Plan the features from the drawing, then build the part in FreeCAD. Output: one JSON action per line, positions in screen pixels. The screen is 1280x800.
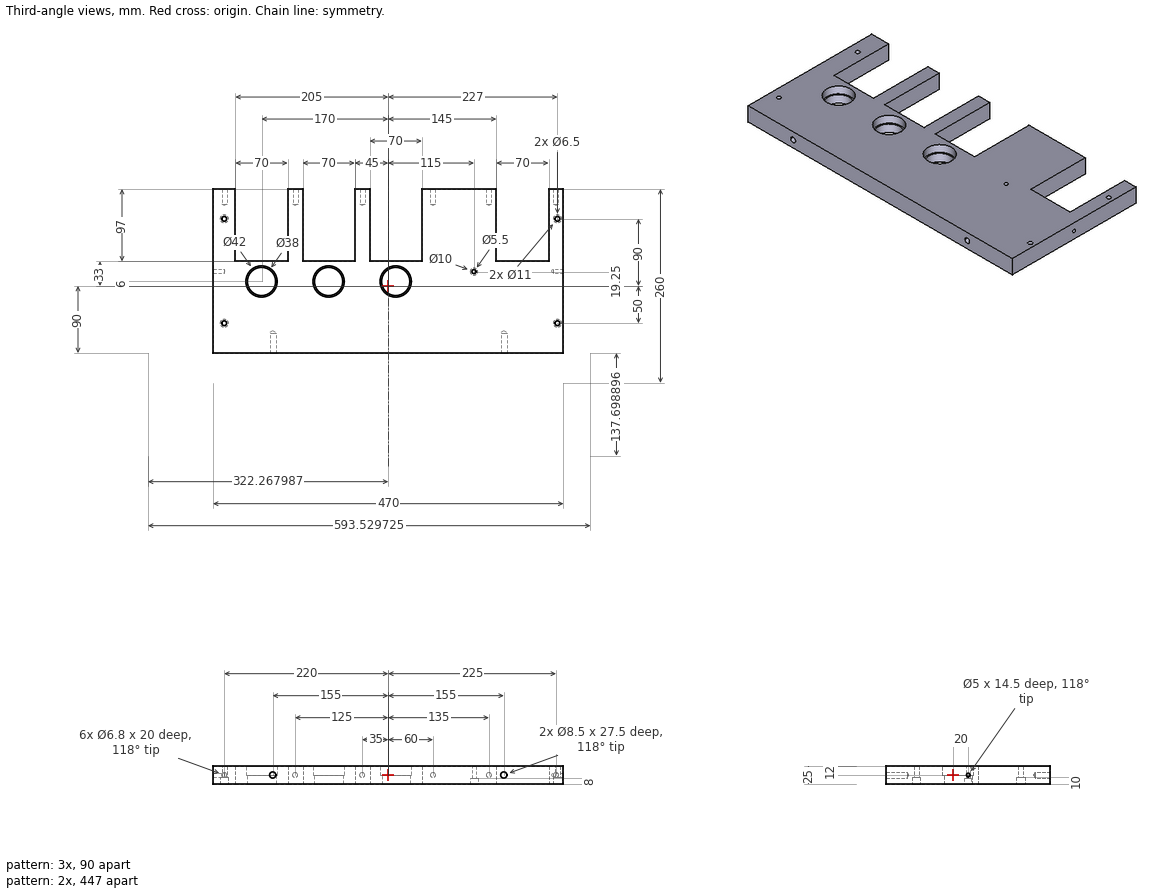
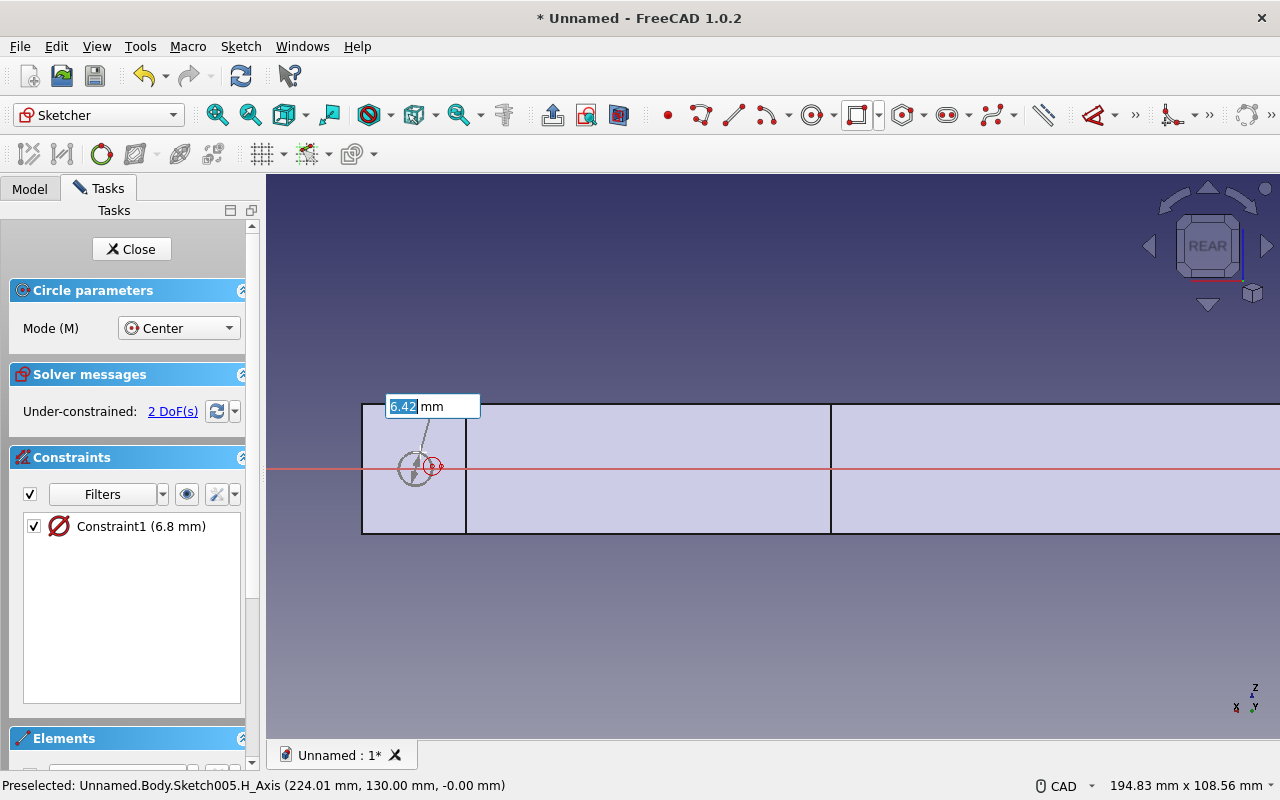
{"action": "type", "text": "6.8"}
{"action": "key", "text": "Return"}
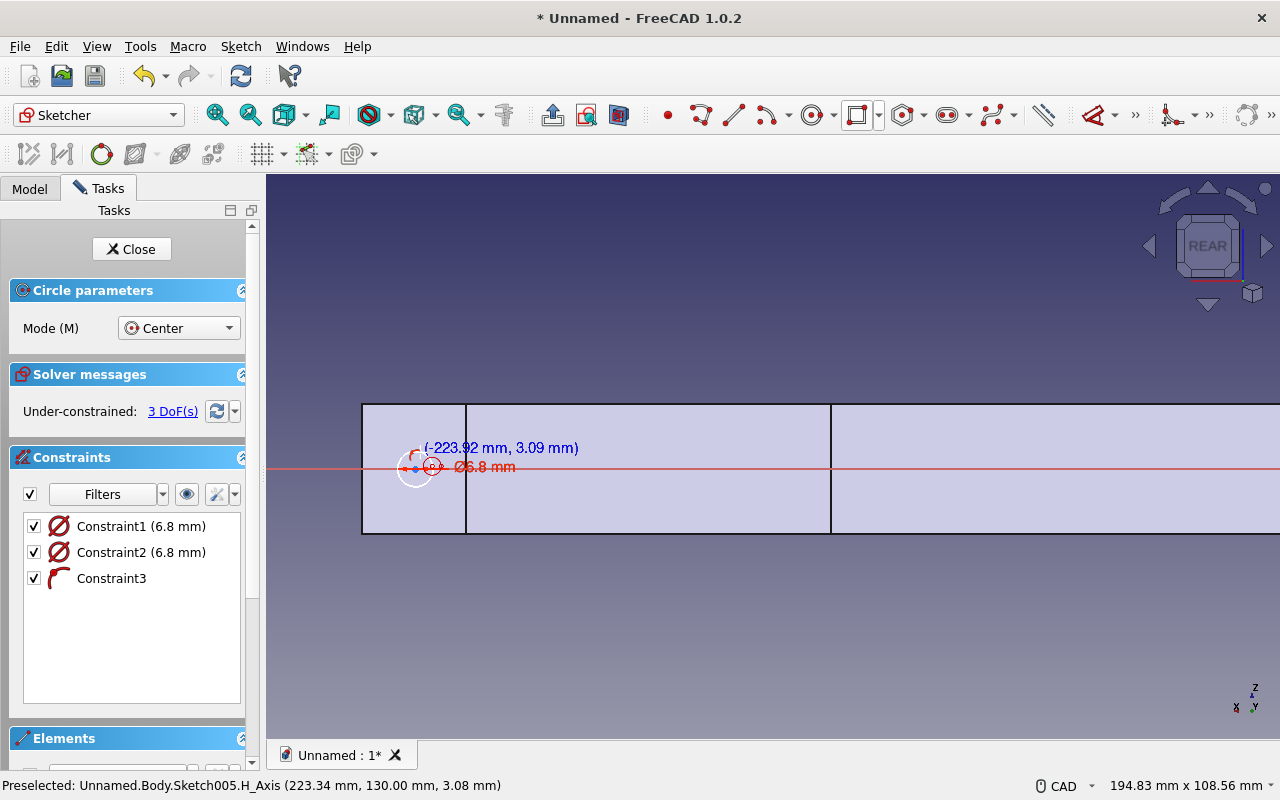
{"action": "scroll", "coordinate": [883, 469], "scroll_direction": "up", "scroll_amount": 2}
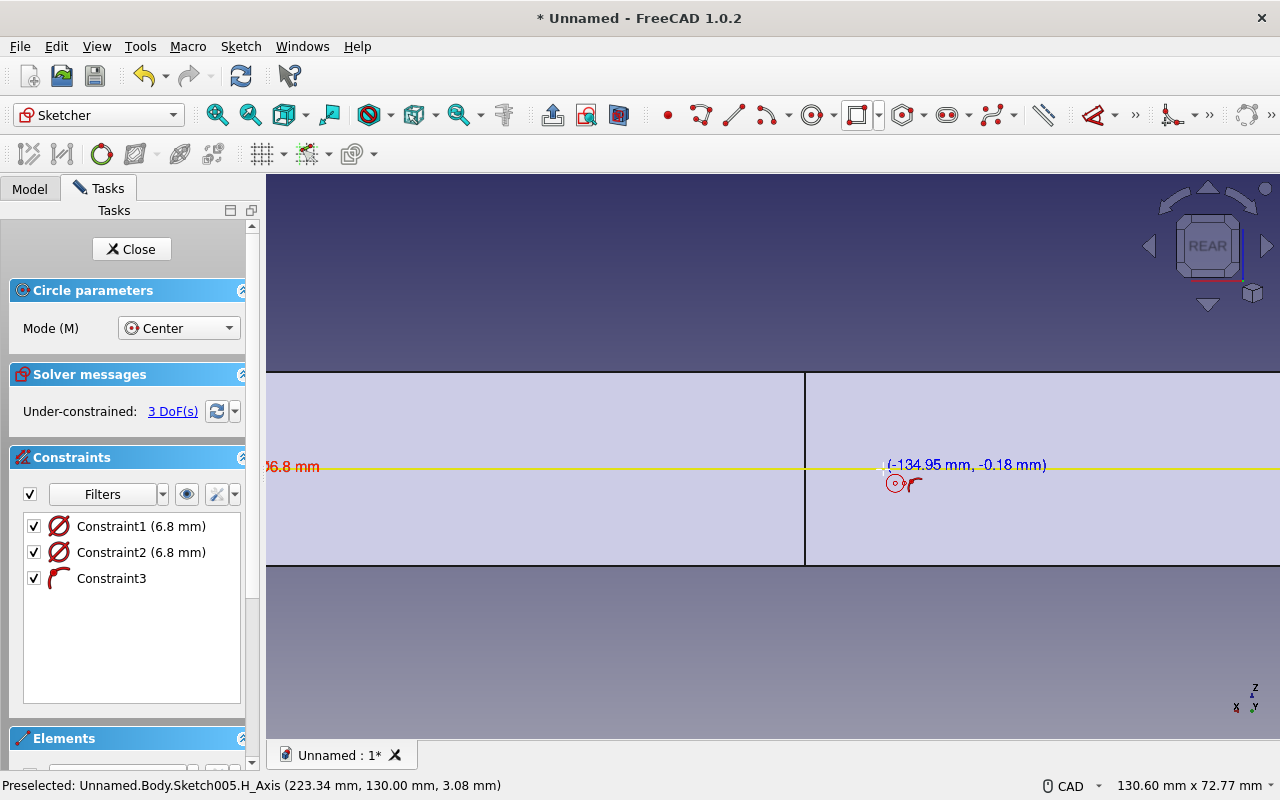
{"action": "scroll", "coordinate": [466, 454], "scroll_direction": "down", "scroll_amount": 9}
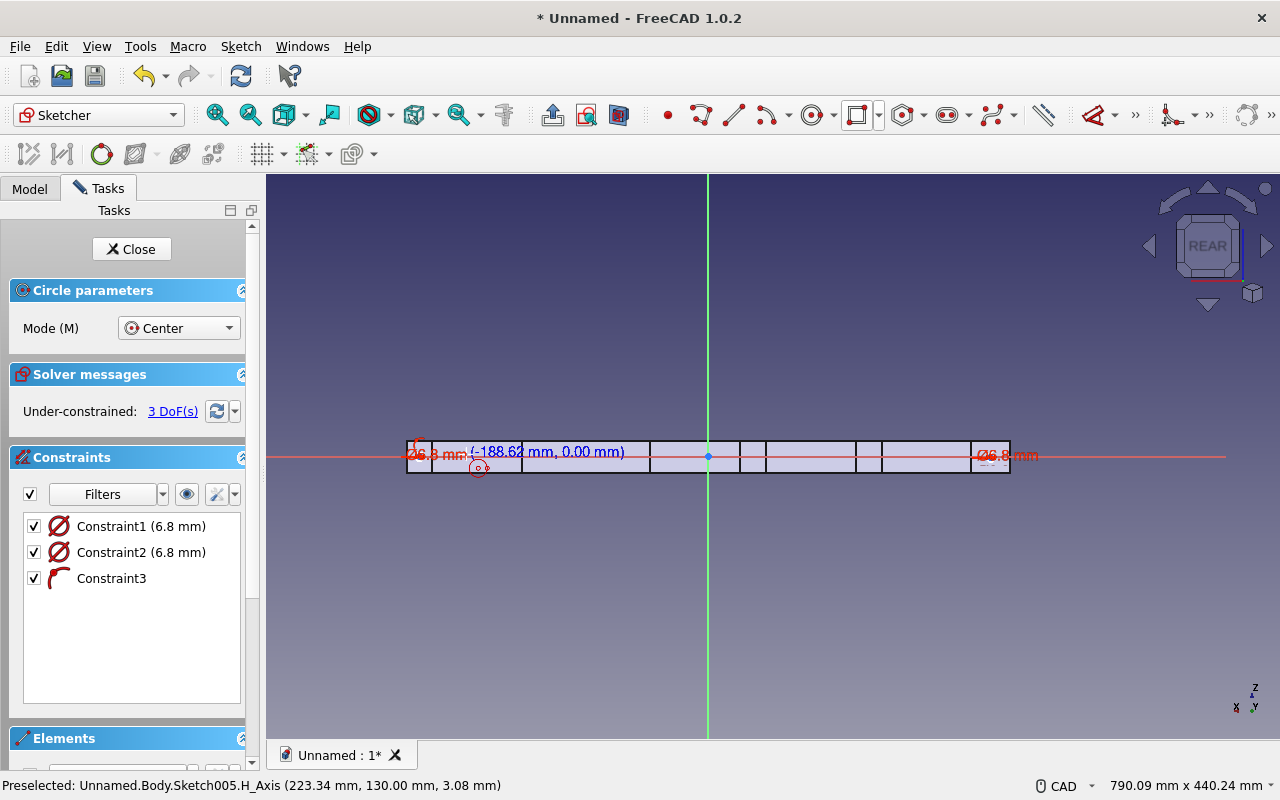
{"action": "left_click", "coordinate": [535, 457]}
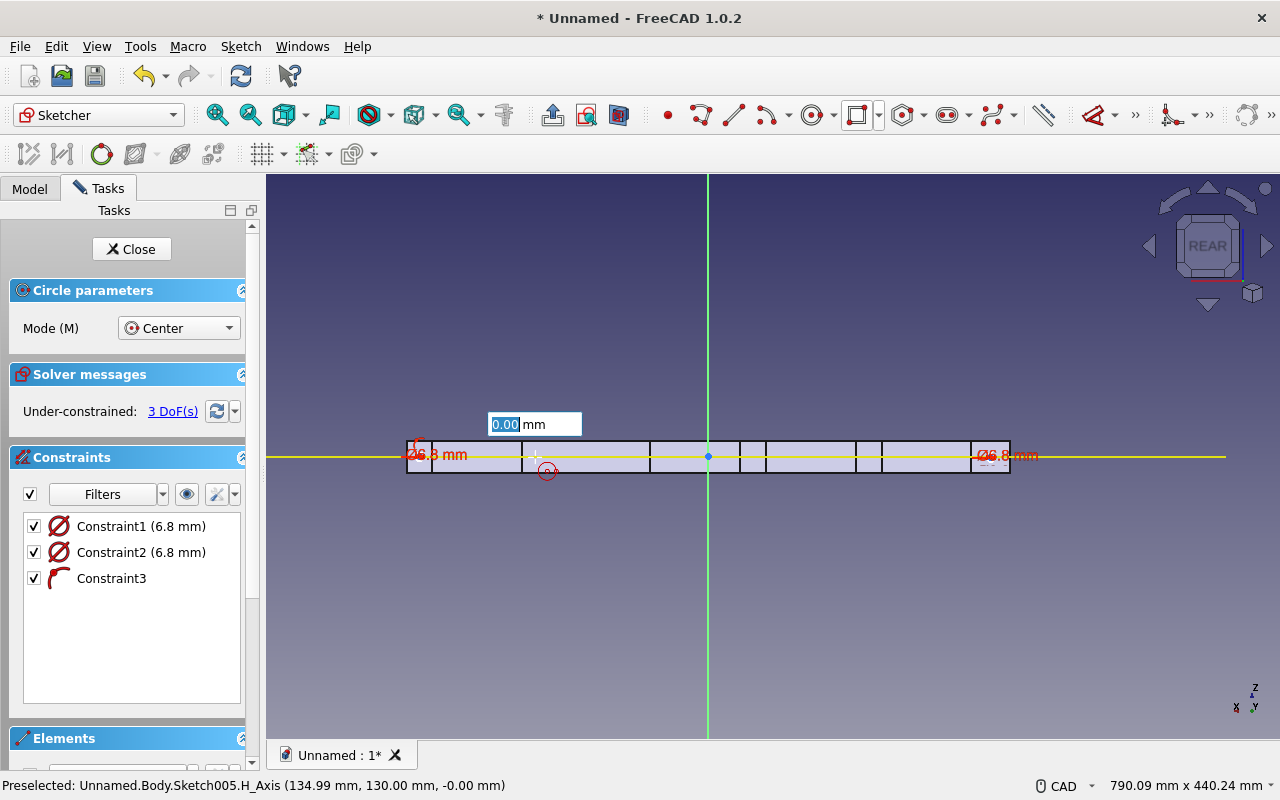
{"action": "scroll", "coordinate": [533, 461], "scroll_direction": "up", "scroll_amount": 7}
{"action": "mouse_move", "coordinate": [534, 459]}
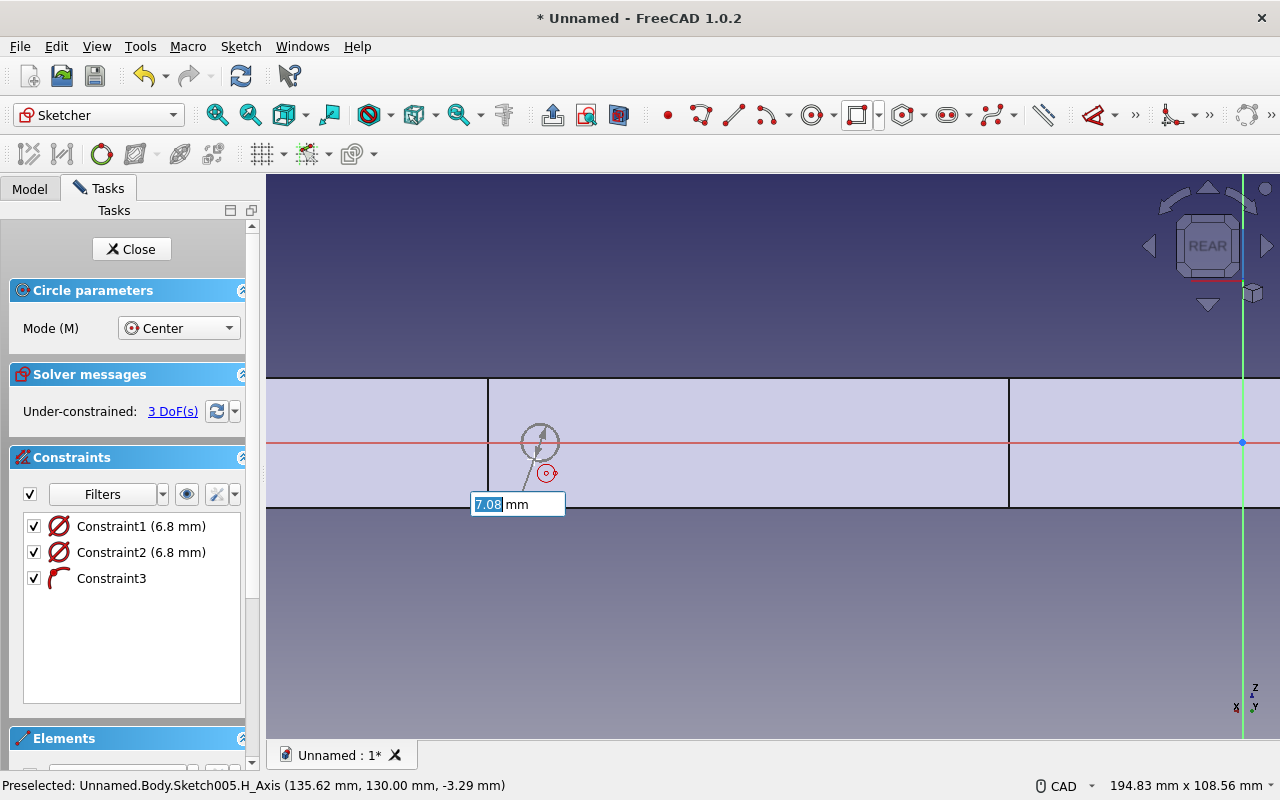
{"action": "type", "text": "6.8"}
{"action": "key", "text": "Return"}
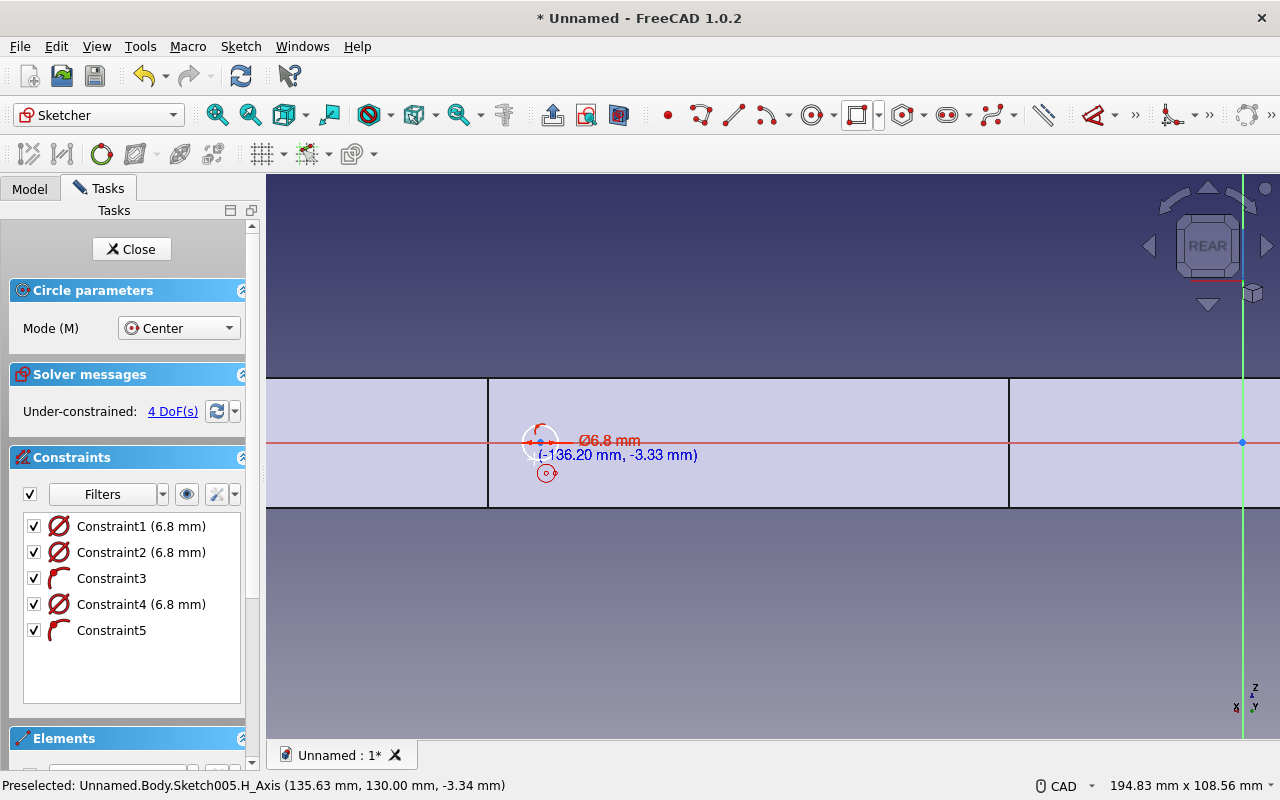
{"action": "scroll", "coordinate": [533, 461], "scroll_direction": "down", "scroll_amount": 7}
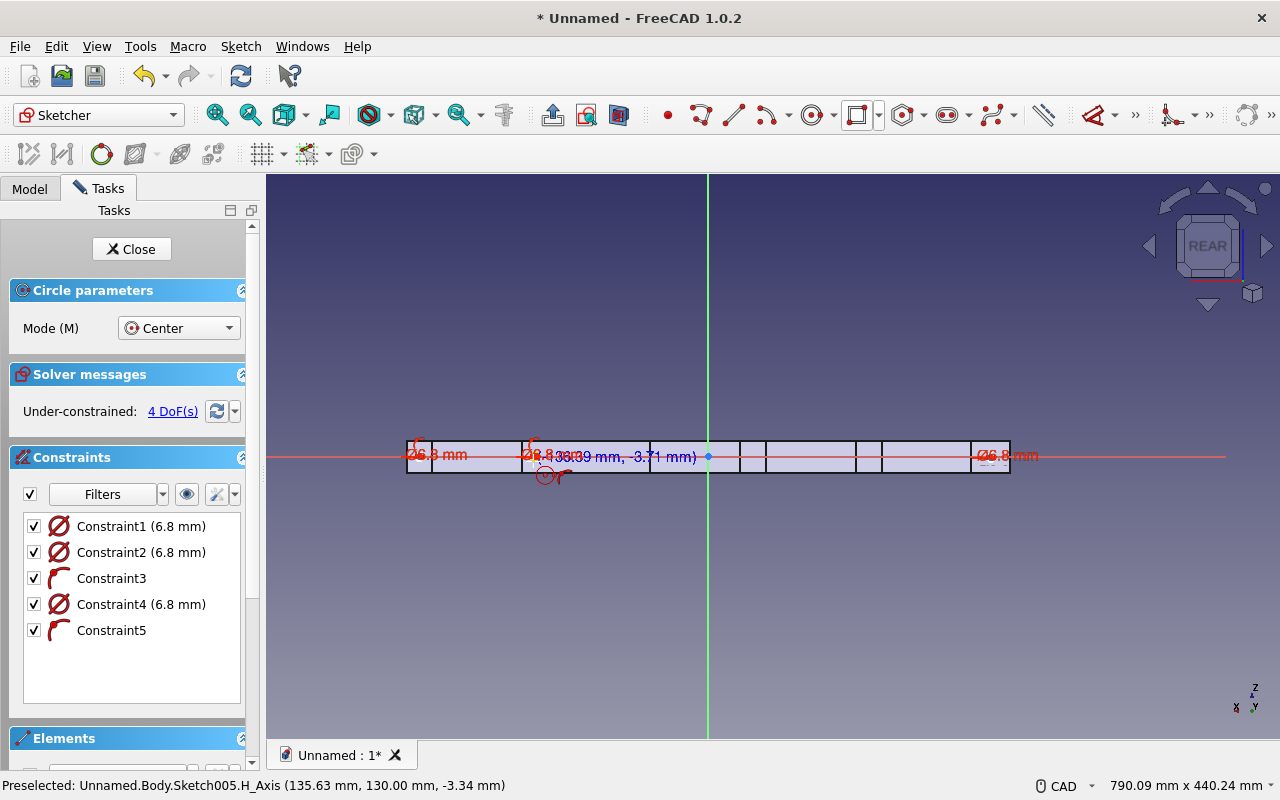
{"action": "scroll", "coordinate": [753, 457], "scroll_direction": "up", "scroll_amount": 9}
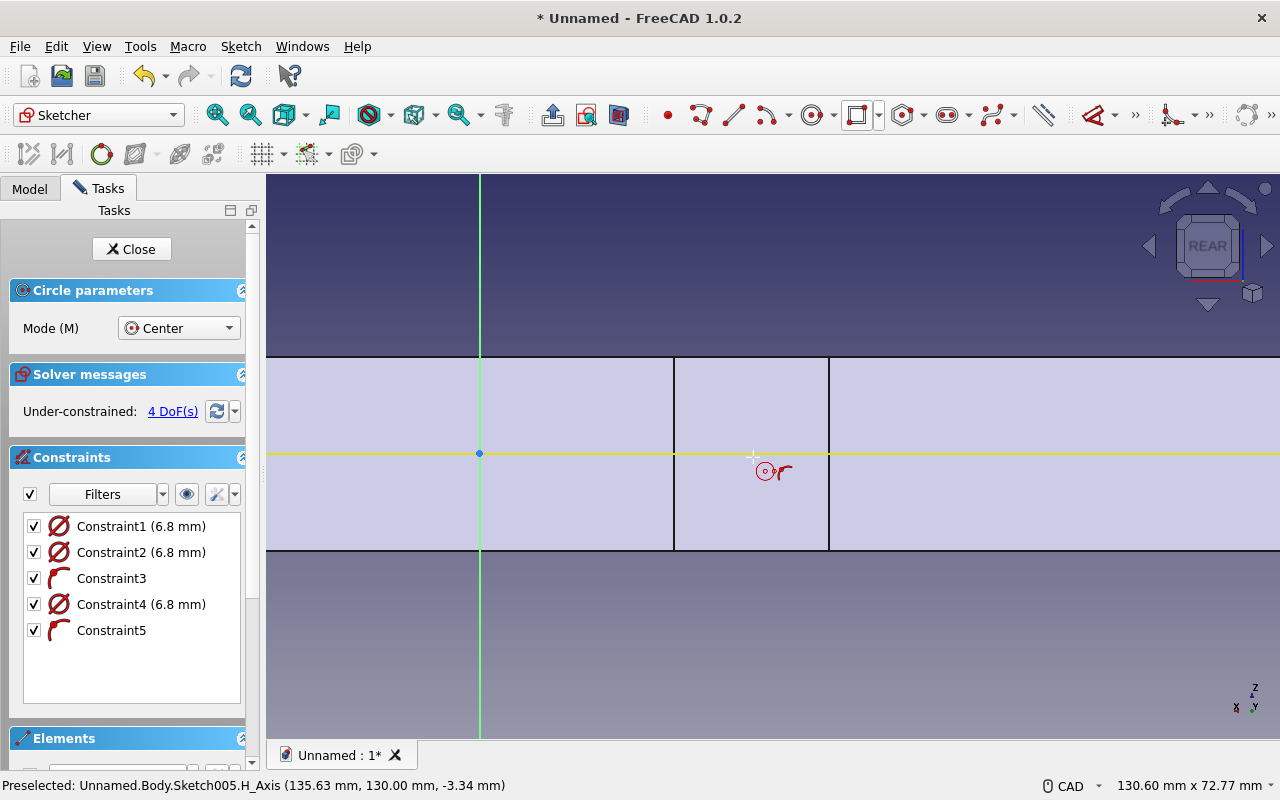
{"action": "scroll", "coordinate": [753, 457], "scroll_direction": "down", "scroll_amount": 9}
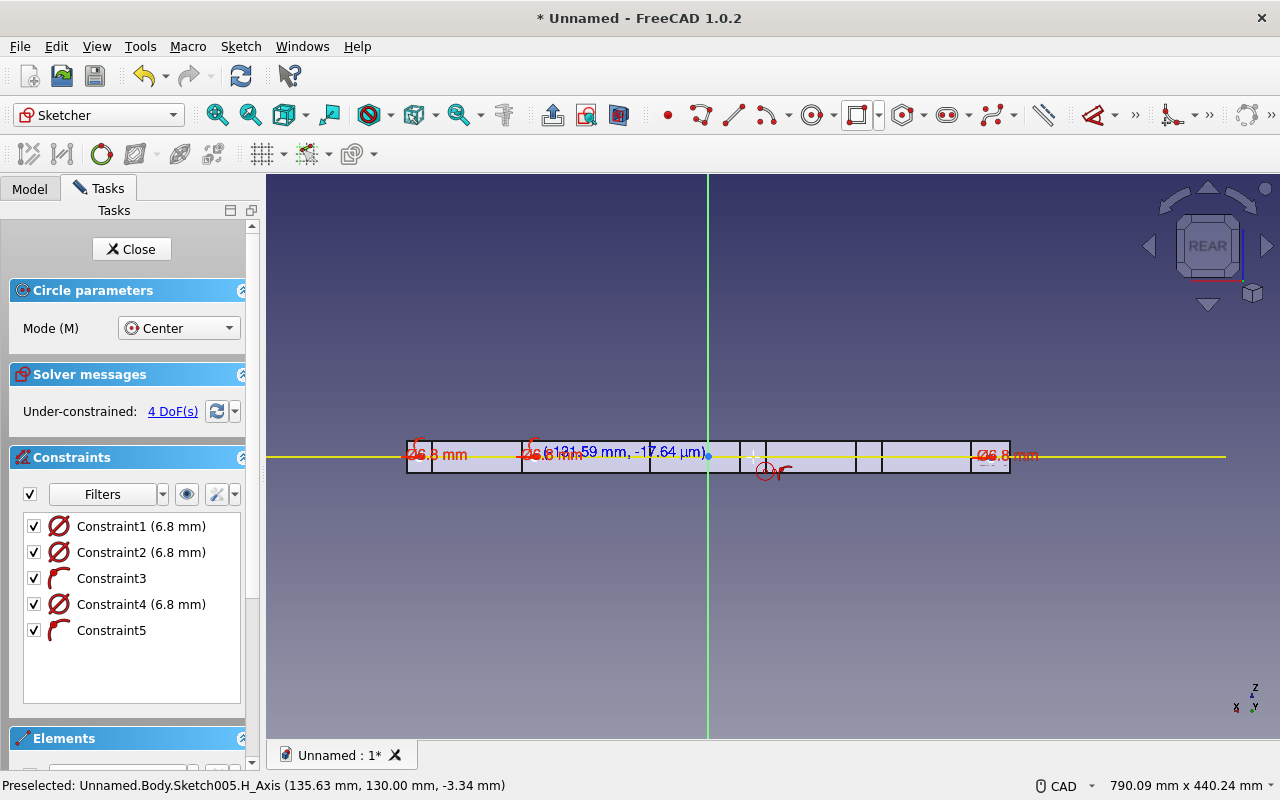
{"action": "left_click", "coordinate": [753, 457]}